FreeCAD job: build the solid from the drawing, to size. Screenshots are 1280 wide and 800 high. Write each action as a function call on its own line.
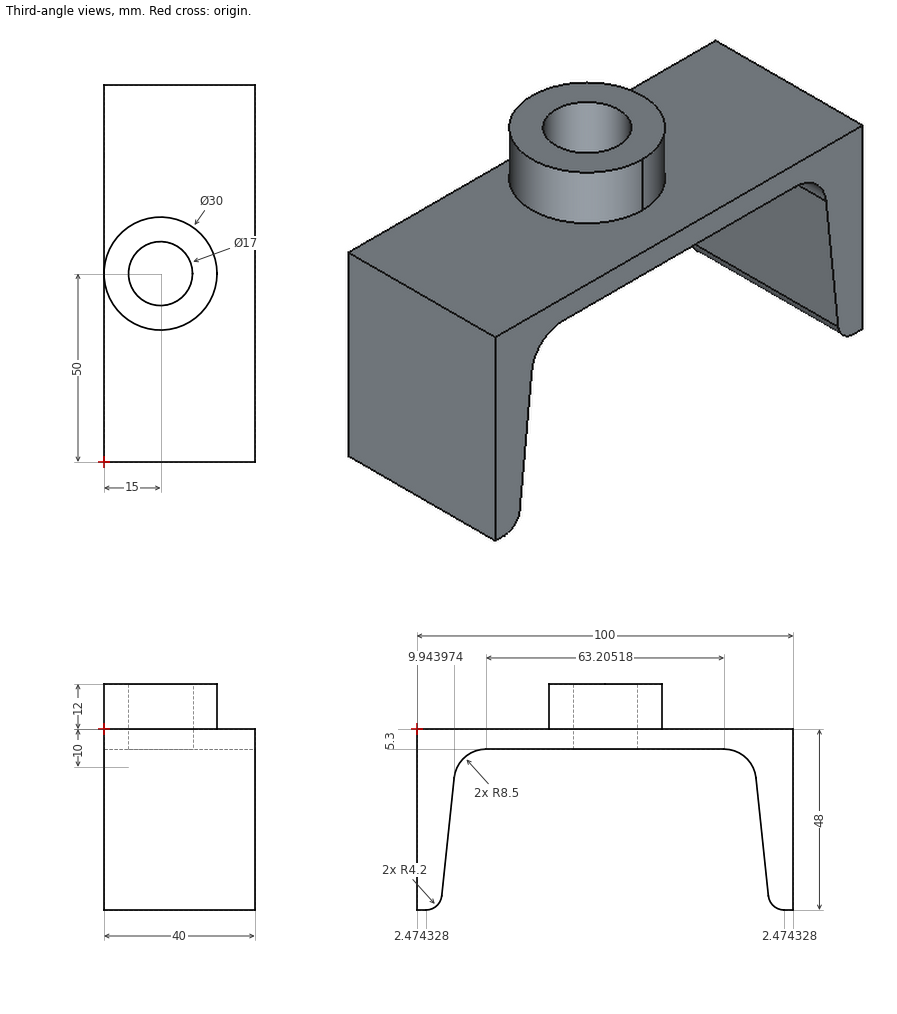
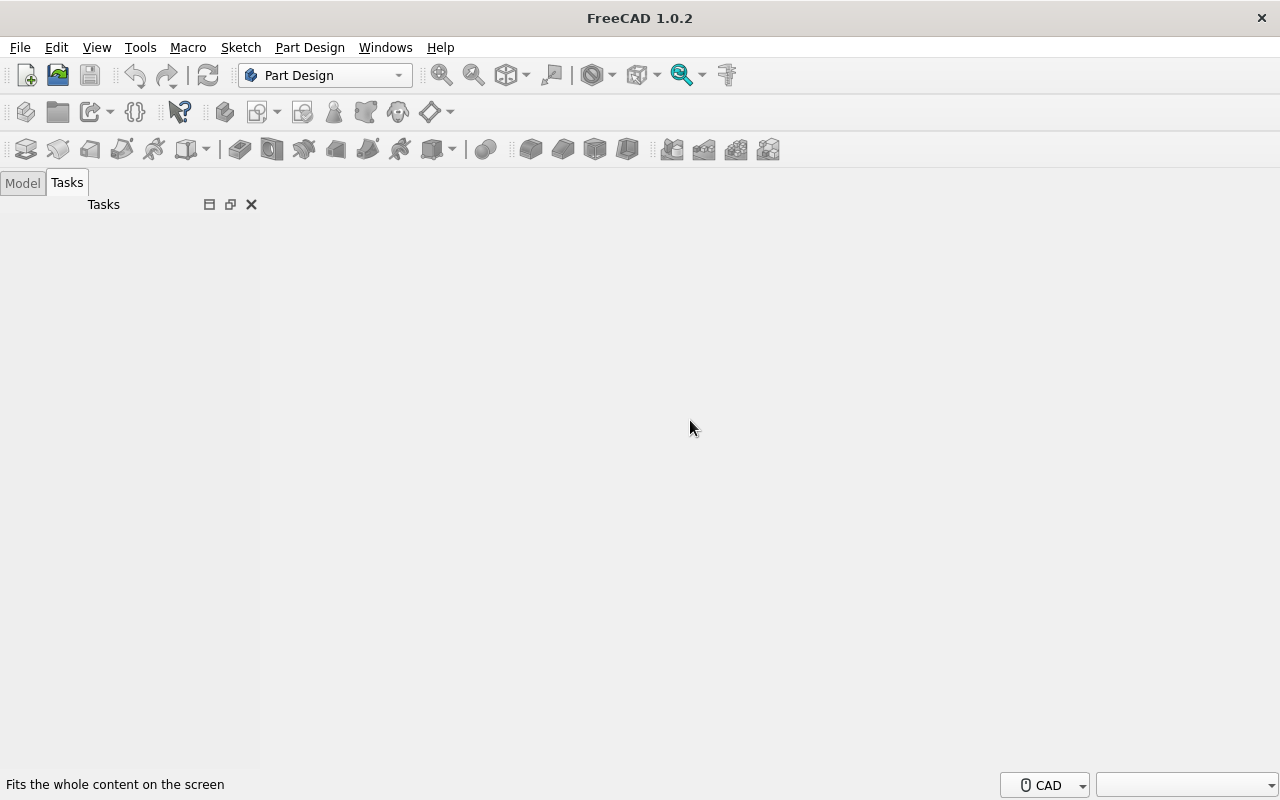
click(26, 76)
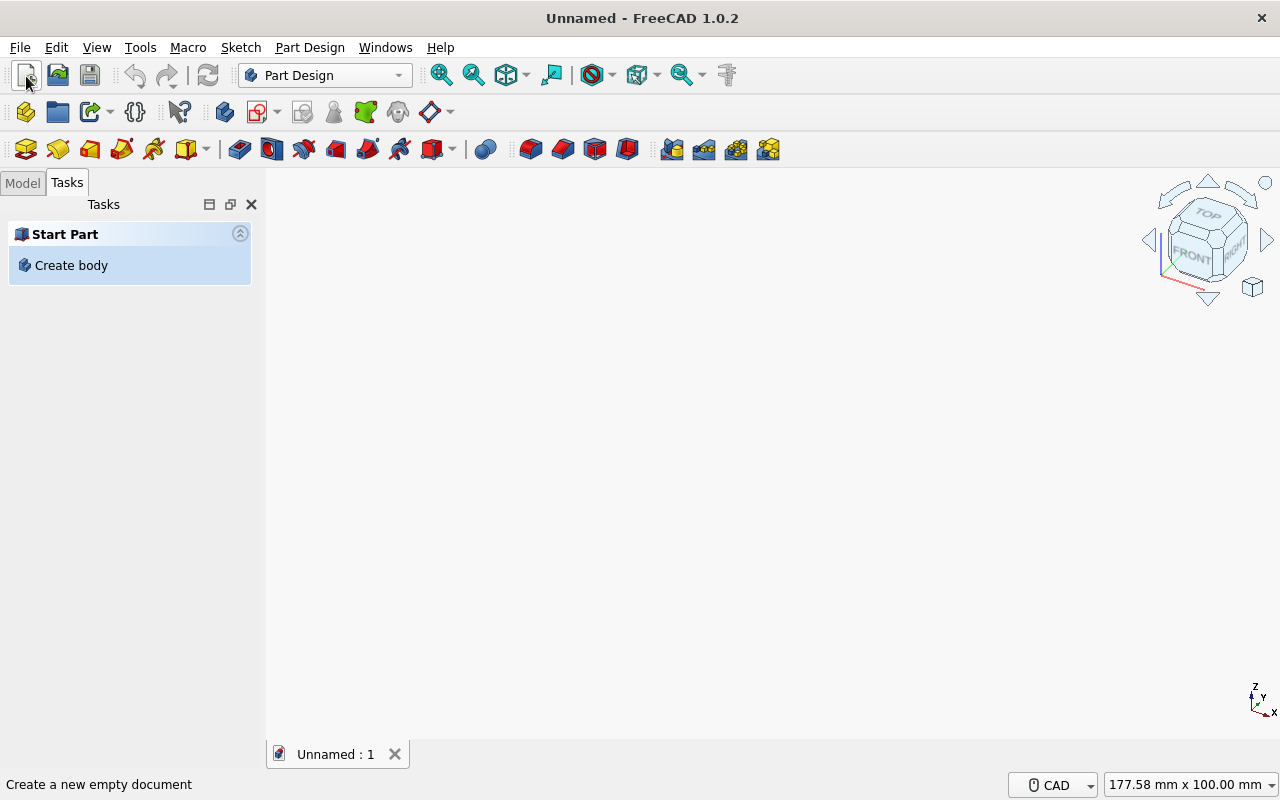
click(258, 112)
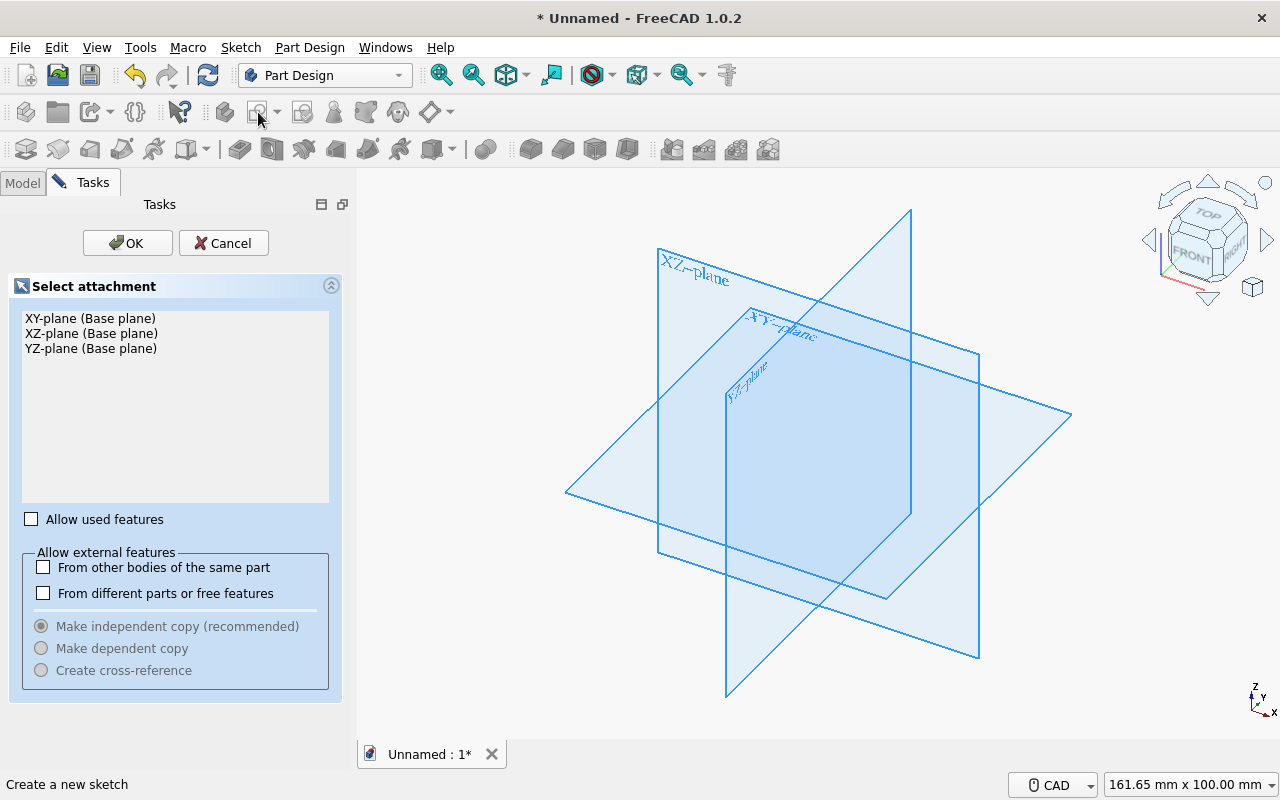
click(82, 348)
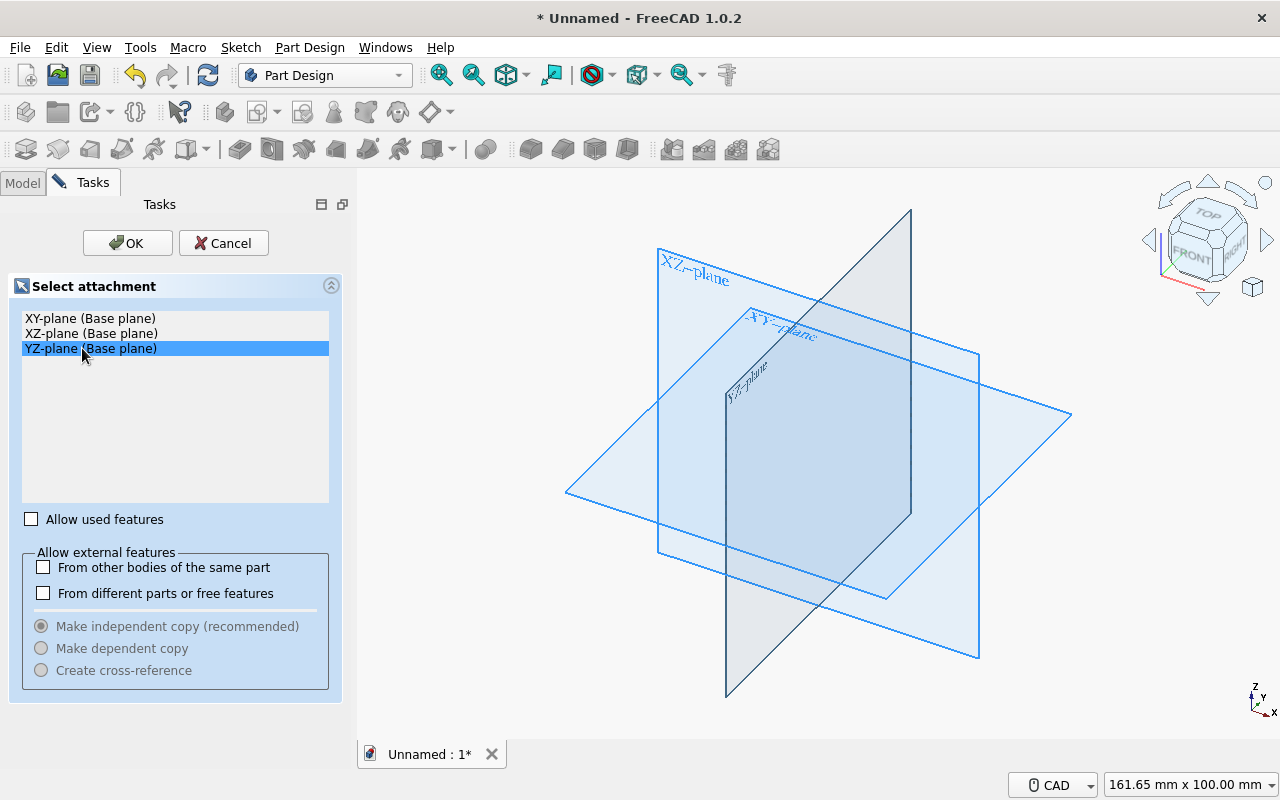
click(128, 243)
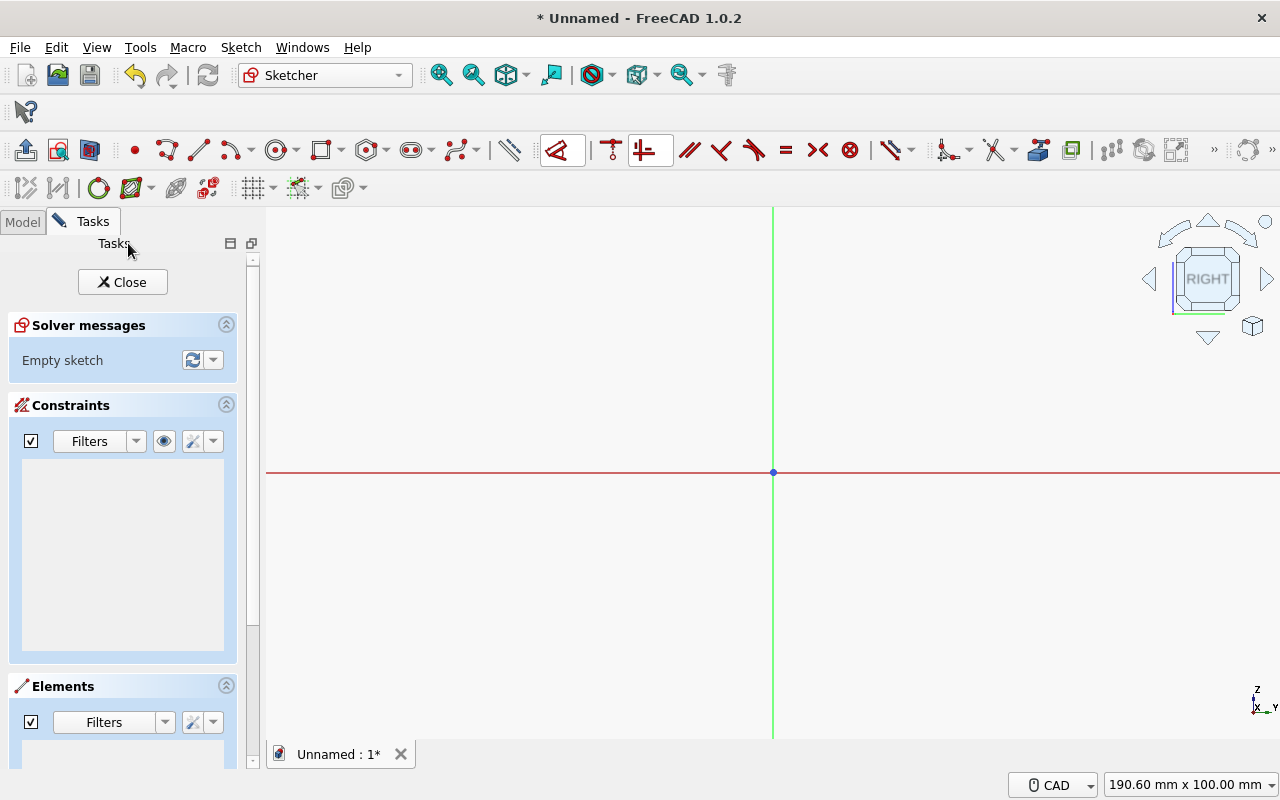
scroll(294, 235, down, 2)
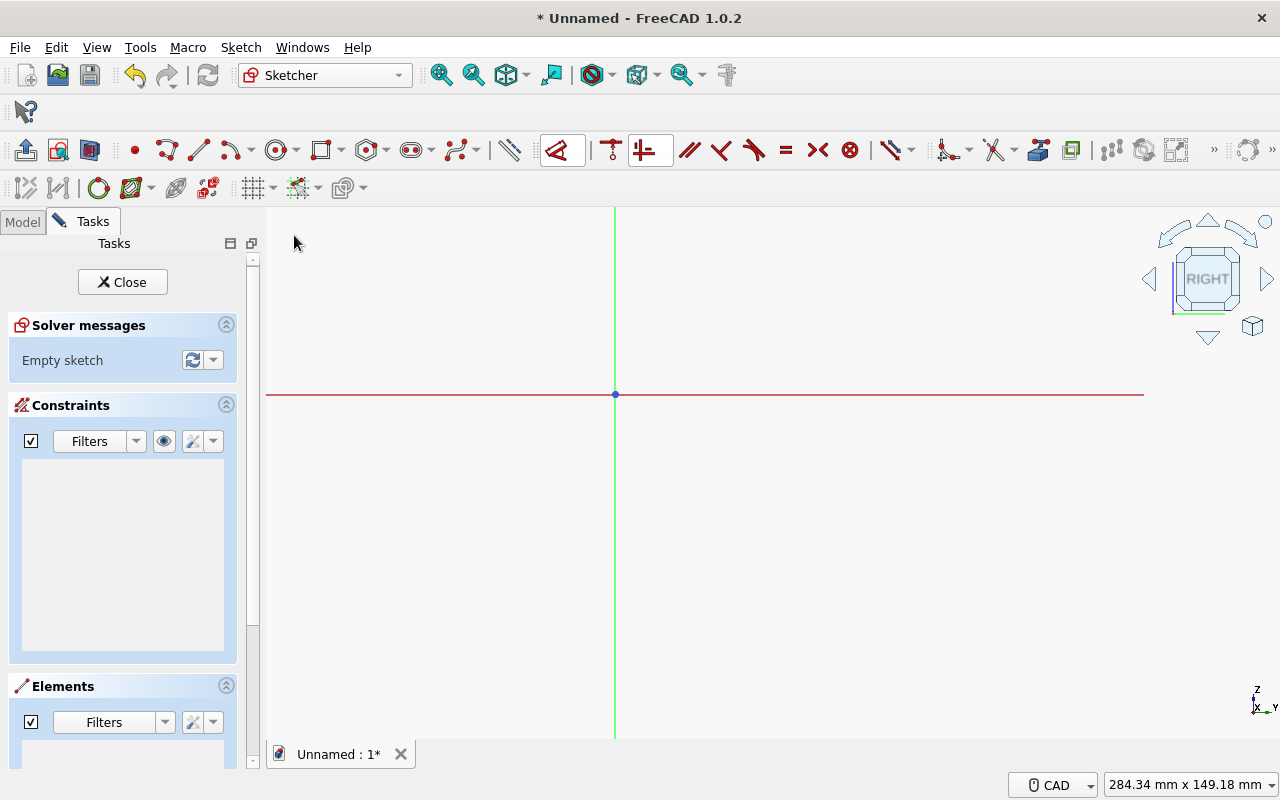
scroll(974, 495, up, 2)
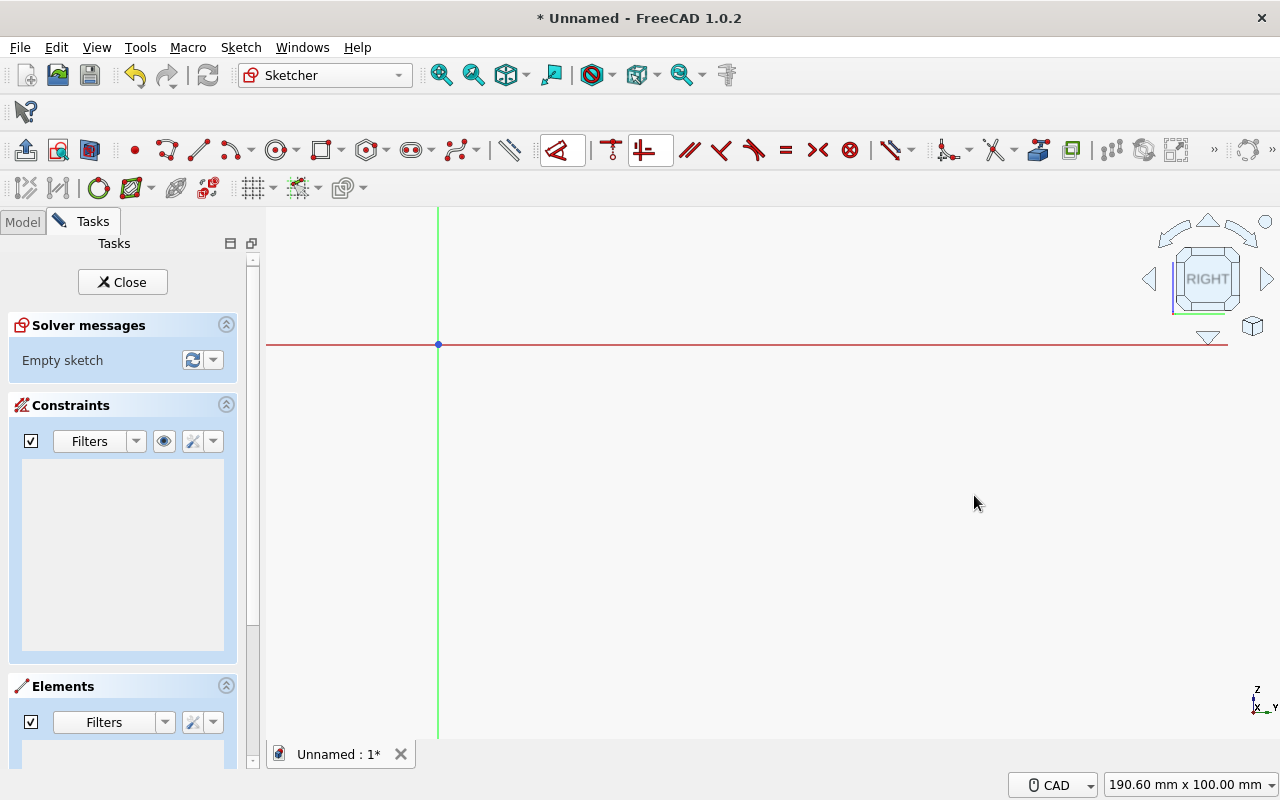
click(200, 150)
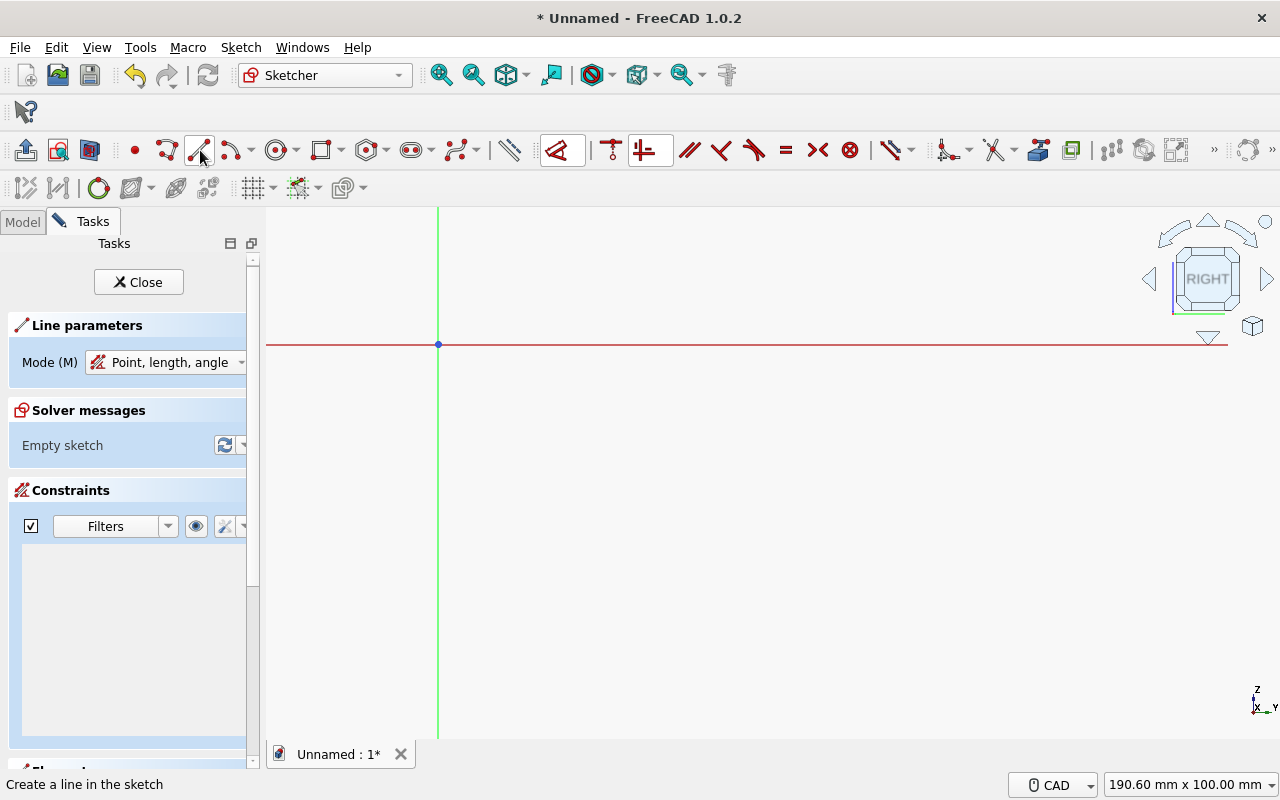
click(474, 580)
click(491, 414)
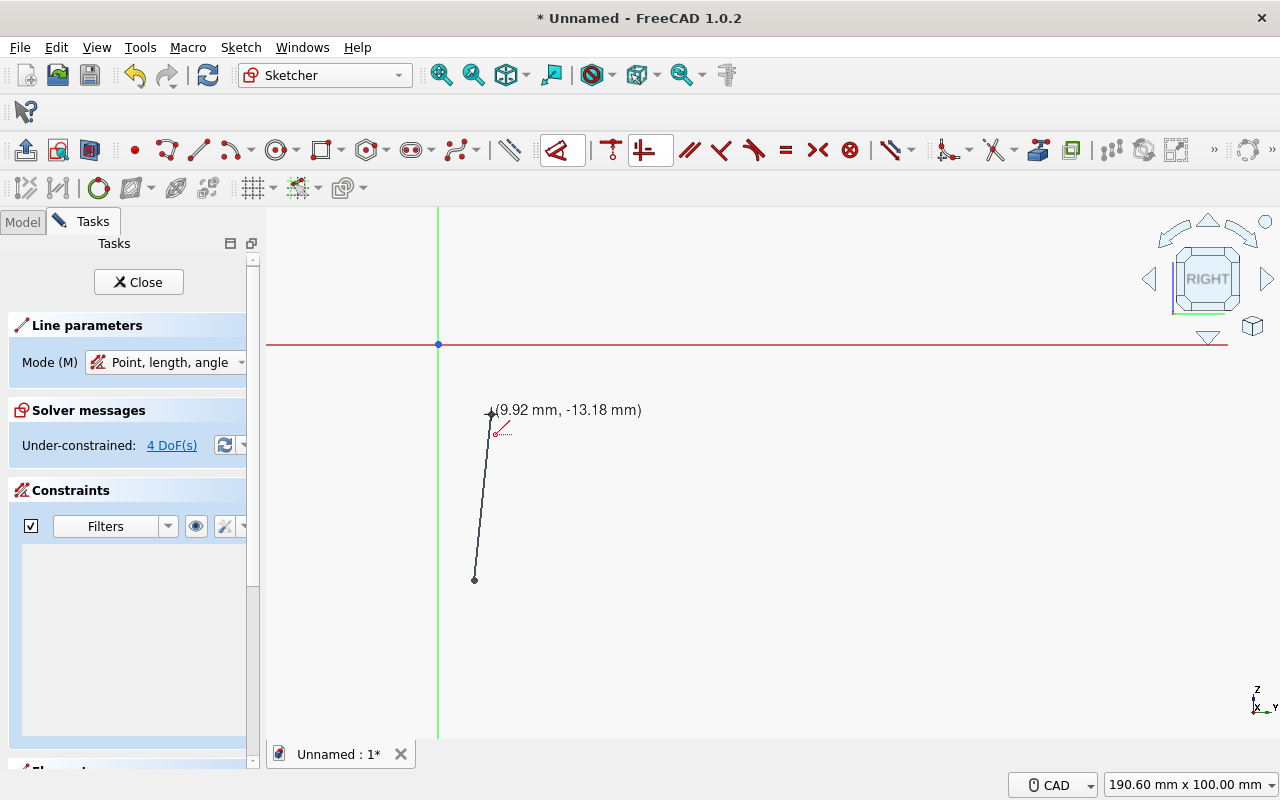
click(536, 373)
click(872, 373)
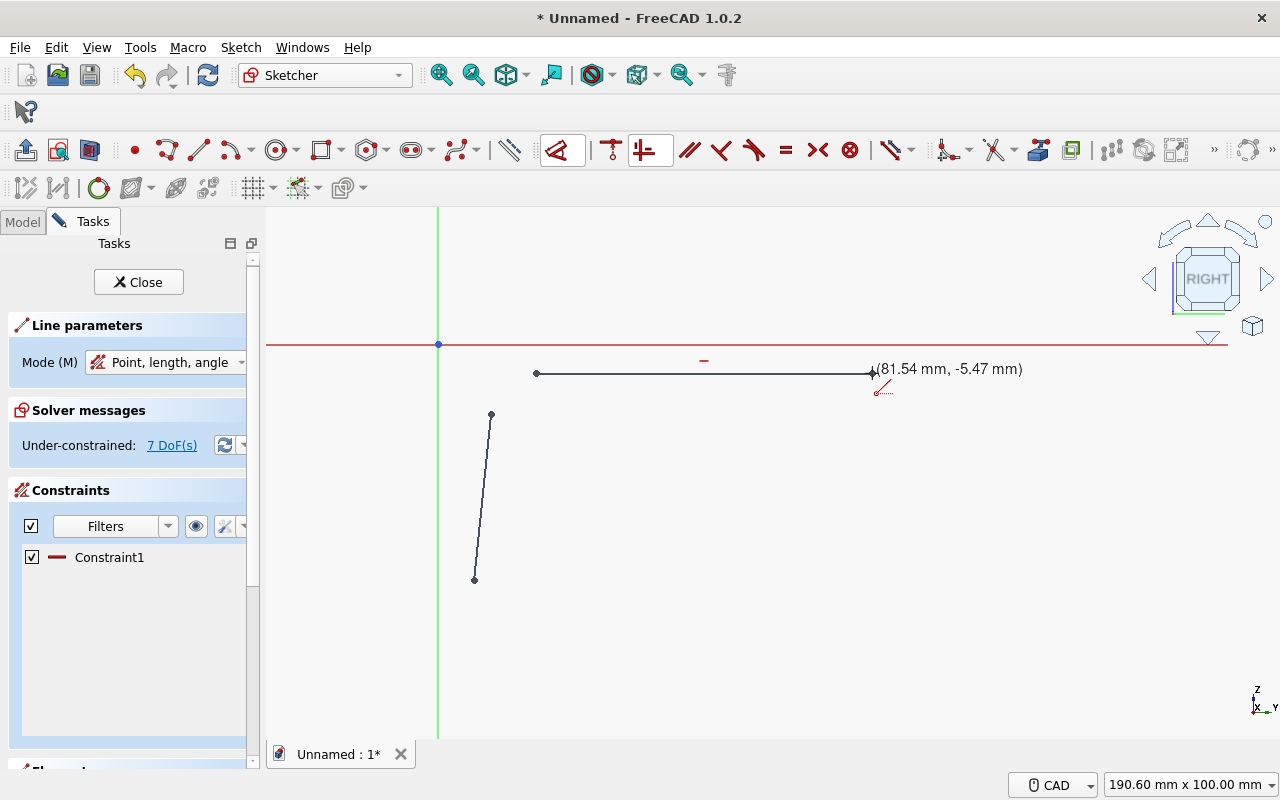
click(917, 414)
click(935, 580)